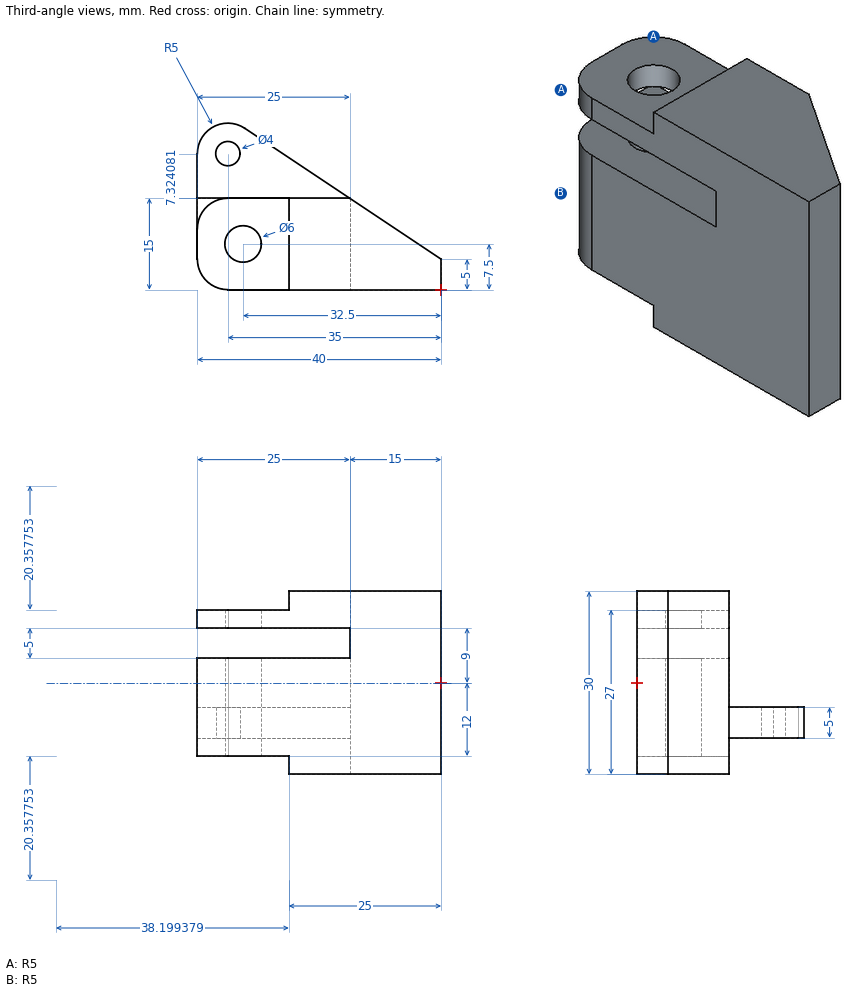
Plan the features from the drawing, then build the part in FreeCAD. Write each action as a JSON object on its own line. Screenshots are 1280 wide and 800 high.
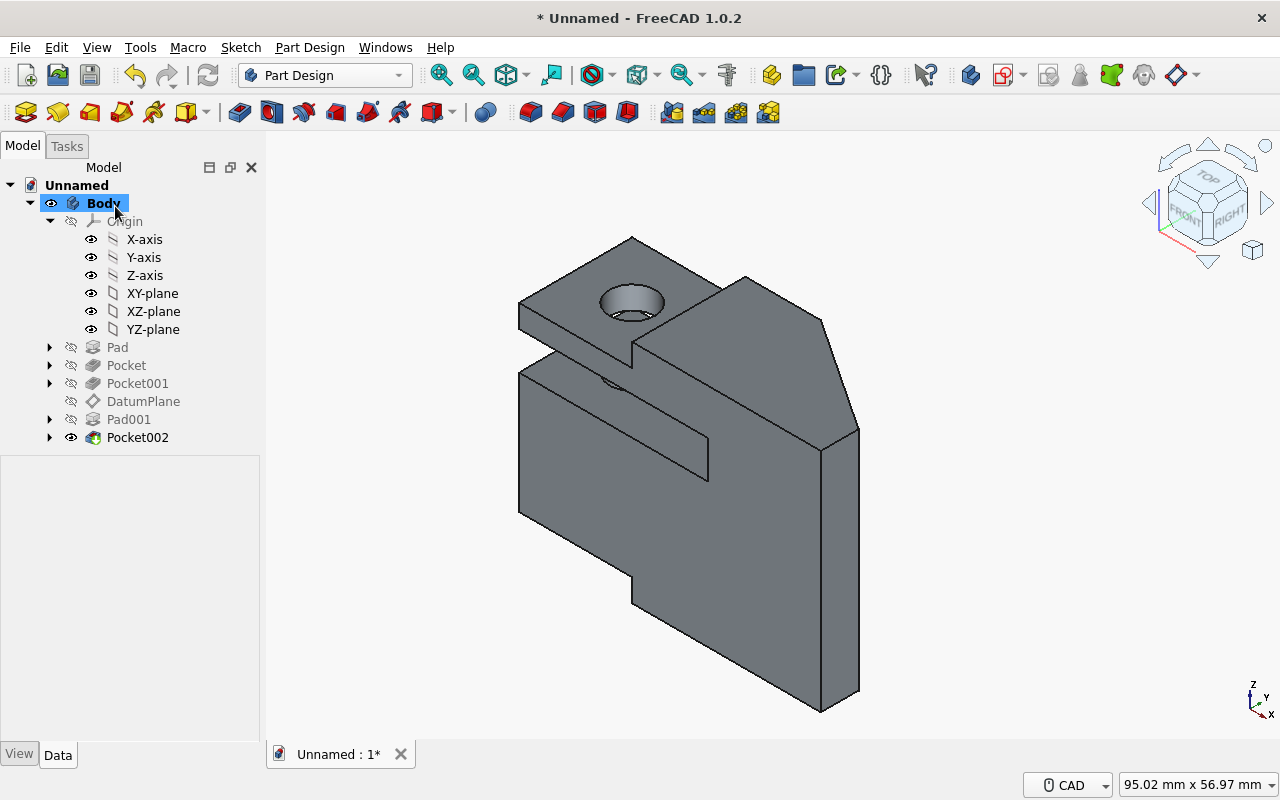
{"action": "key", "text": "2"}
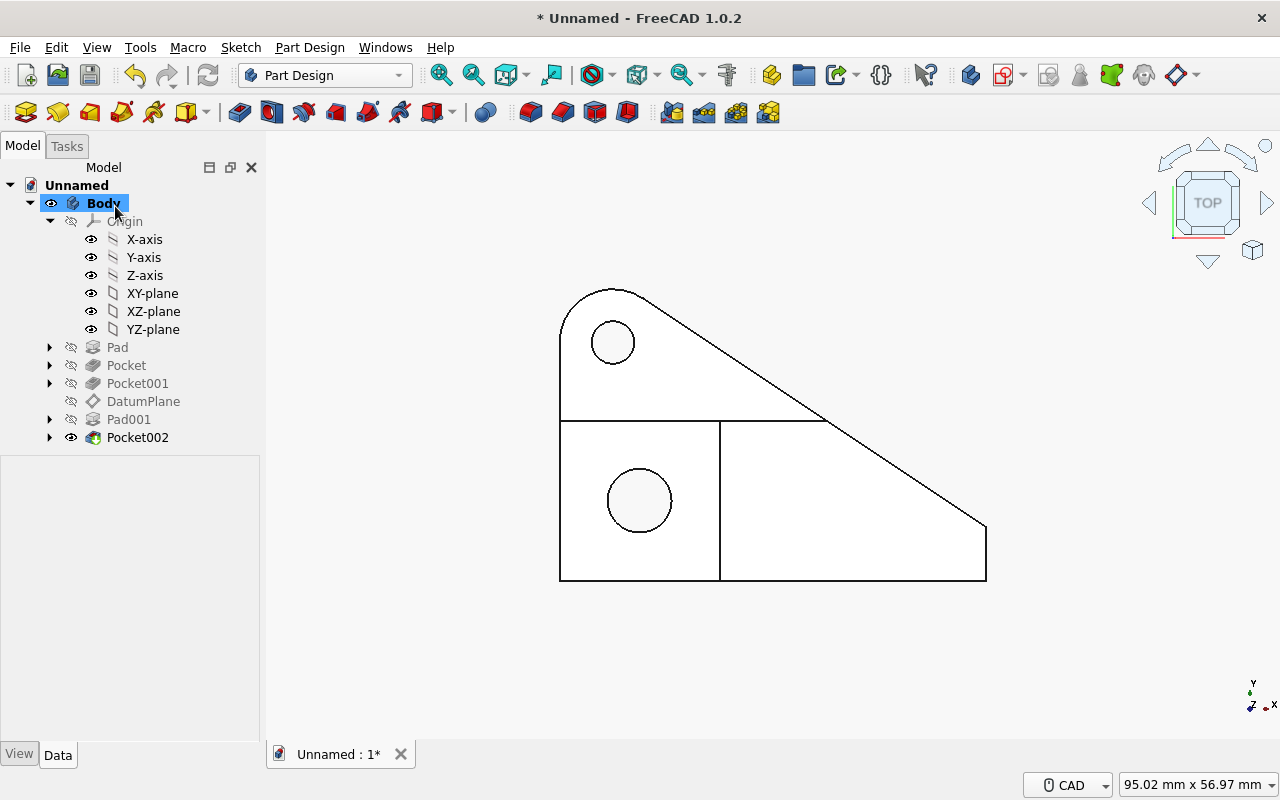
{"action": "key", "text": "0"}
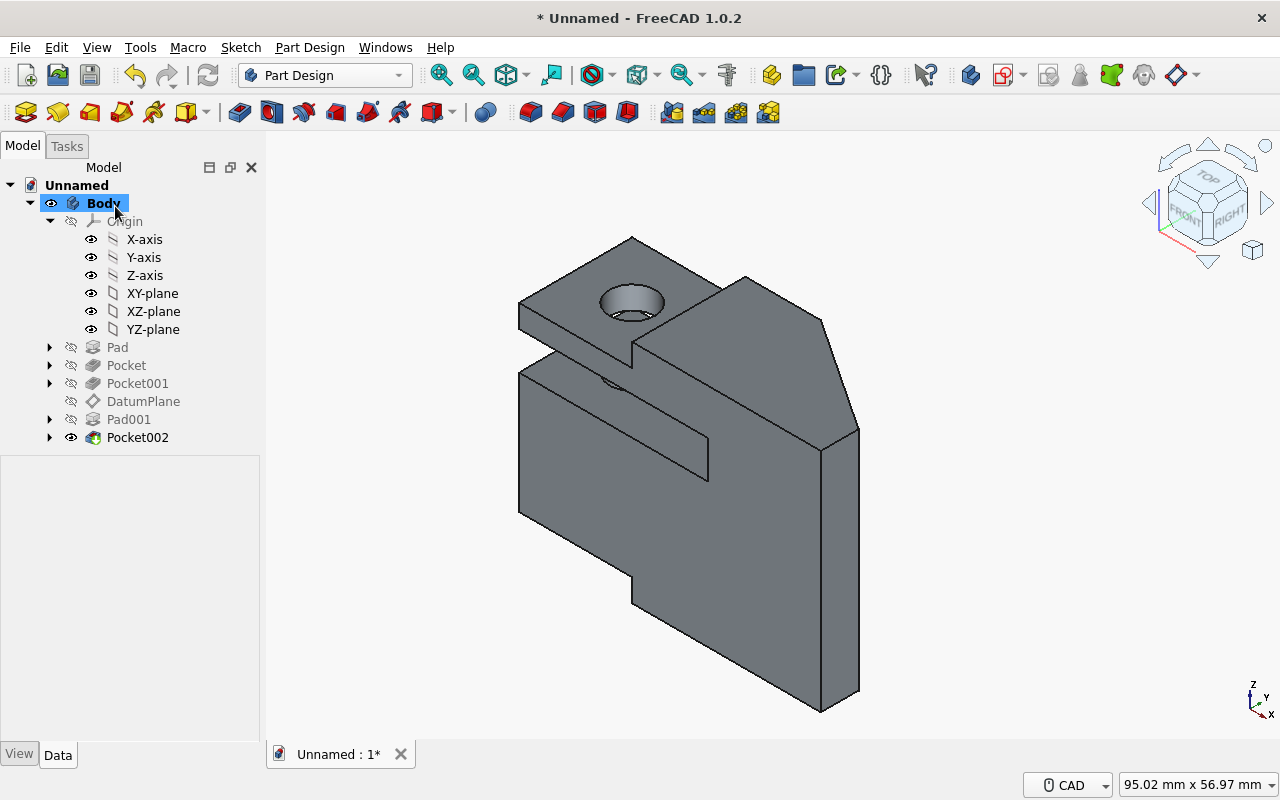
{"action": "key", "text": "1"}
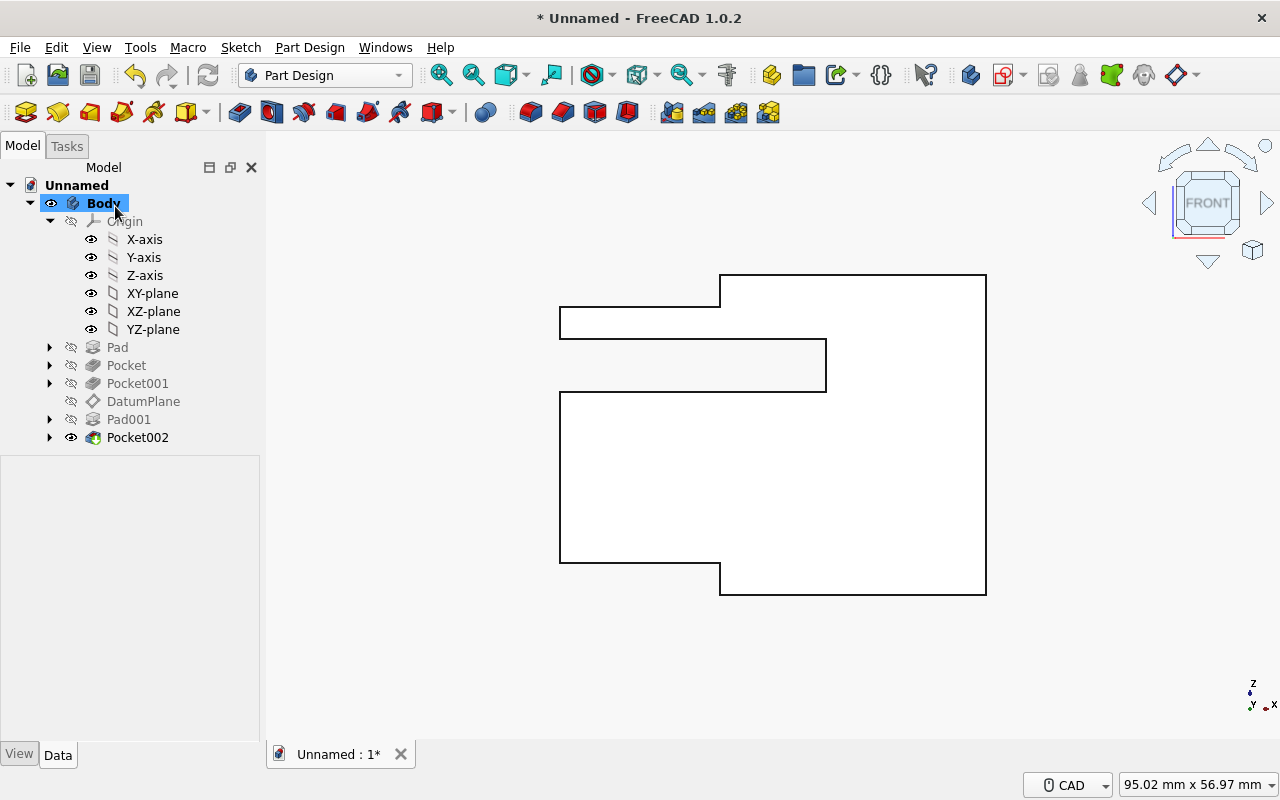
{"action": "left_click", "coordinate": [560, 322]}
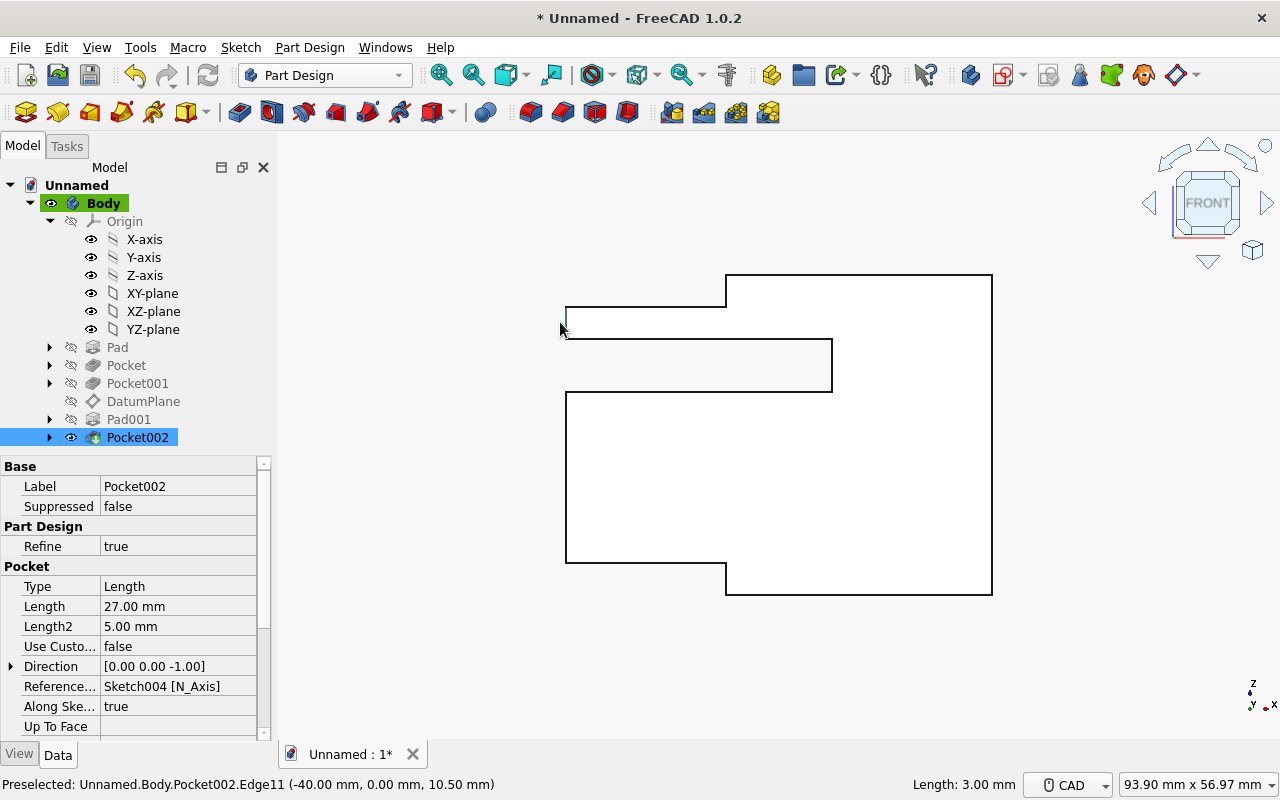
{"action": "key", "text": "3"}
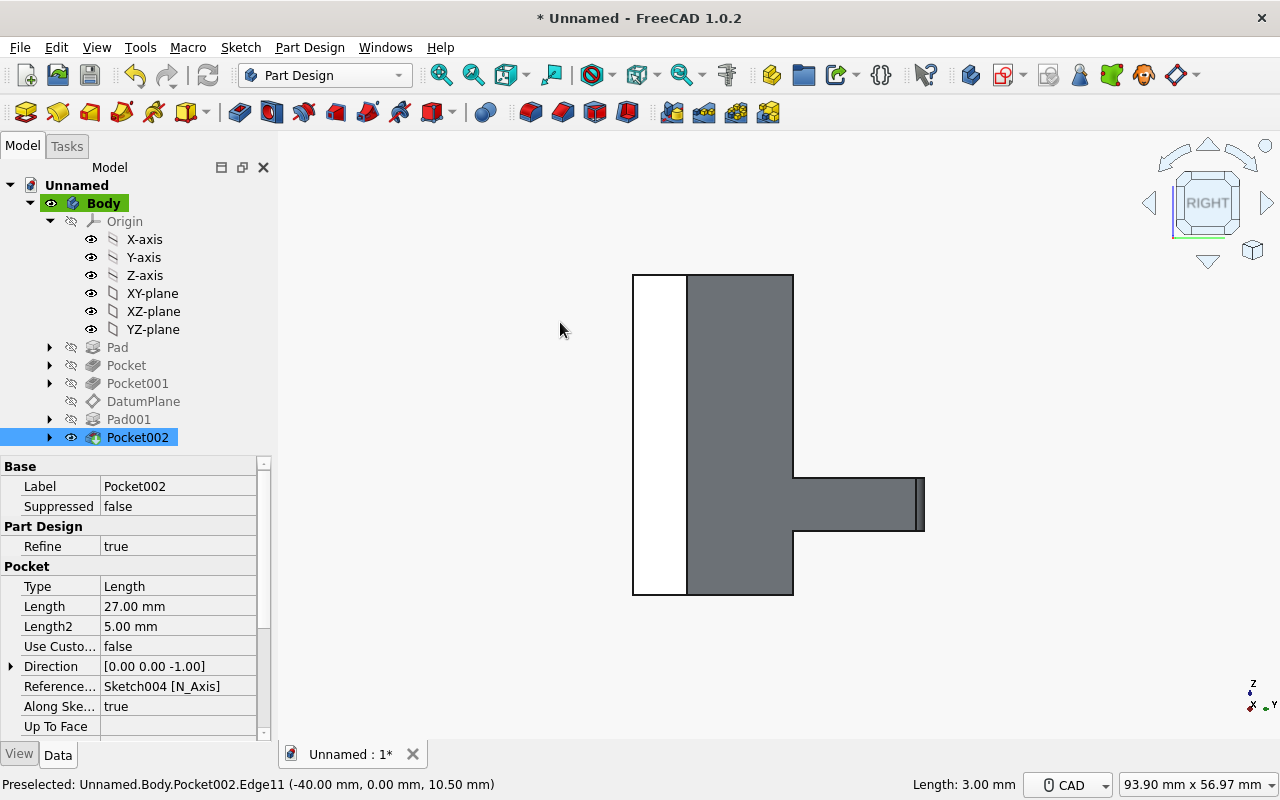
{"action": "key", "text": "5"}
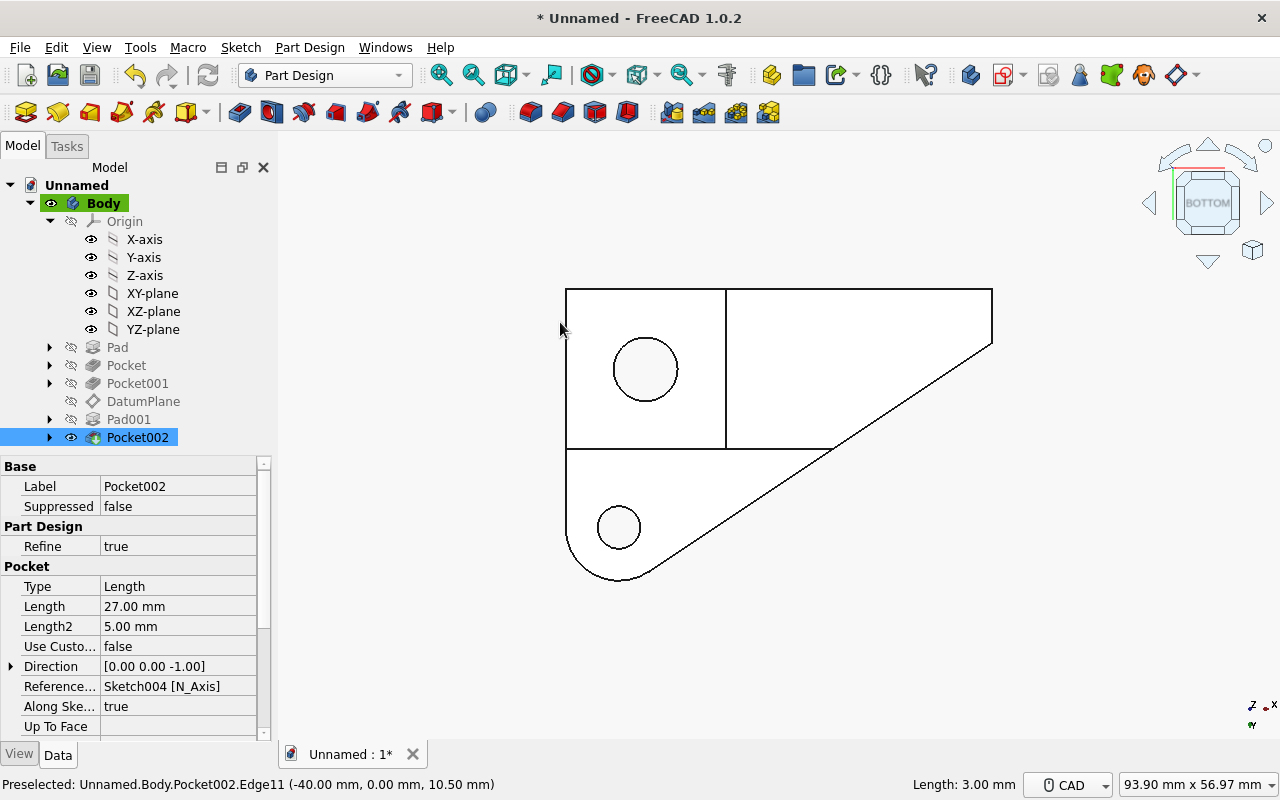
{"action": "key", "text": "4"}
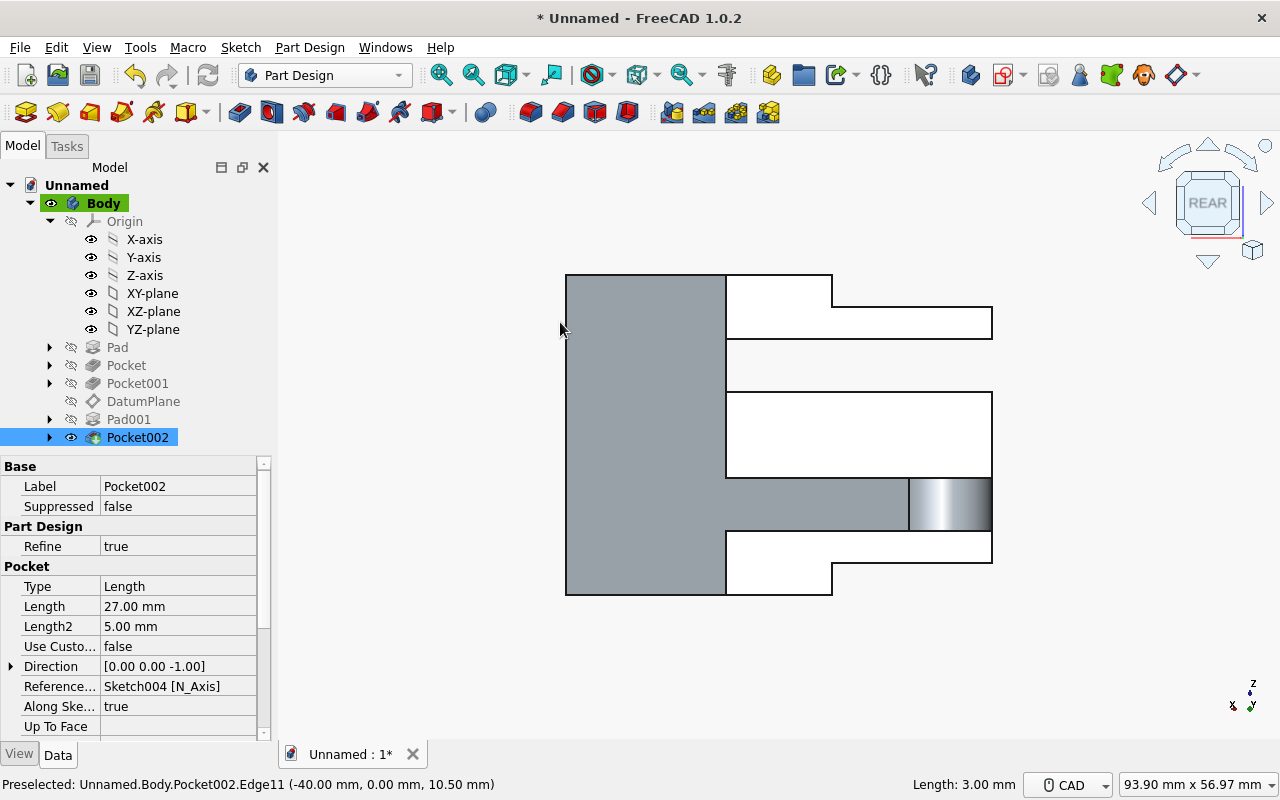
{"action": "left_click", "coordinate": [992, 322], "text": "ctrl"}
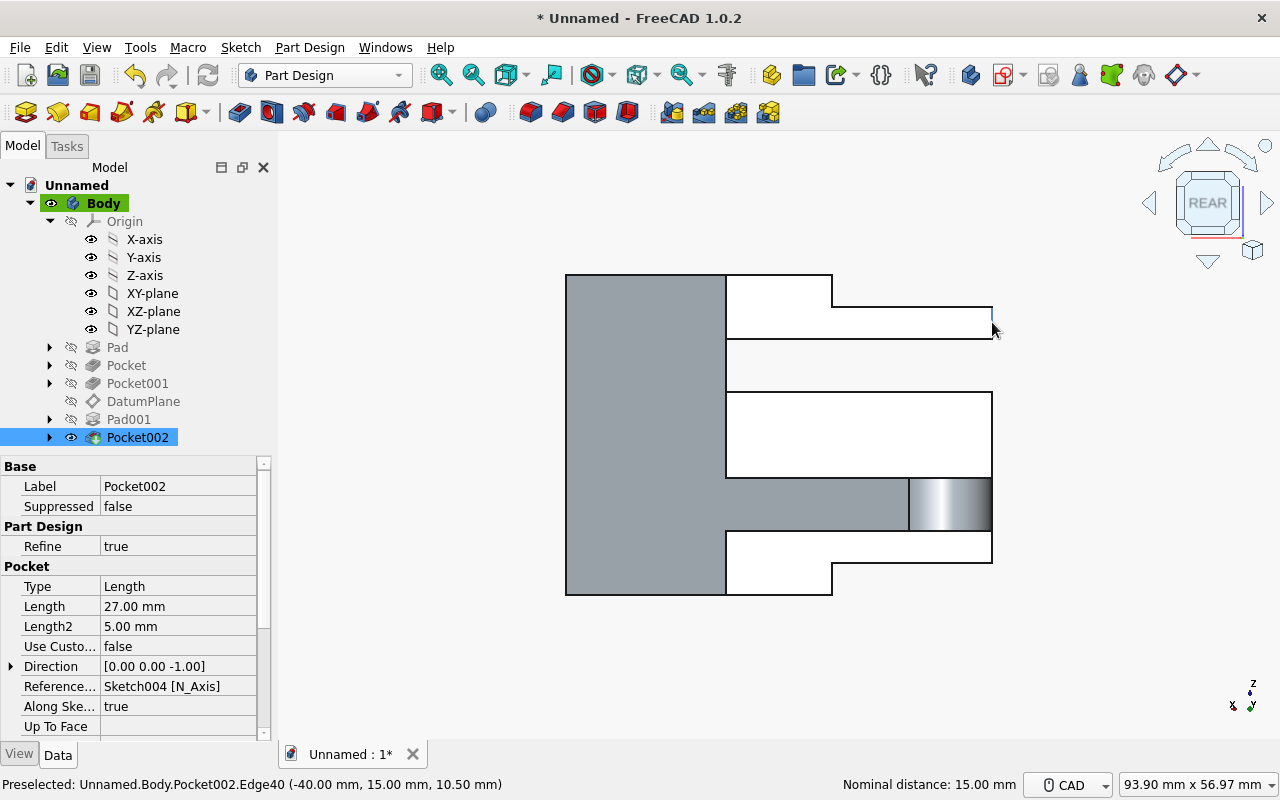
{"action": "left_click", "coordinate": [532, 112]}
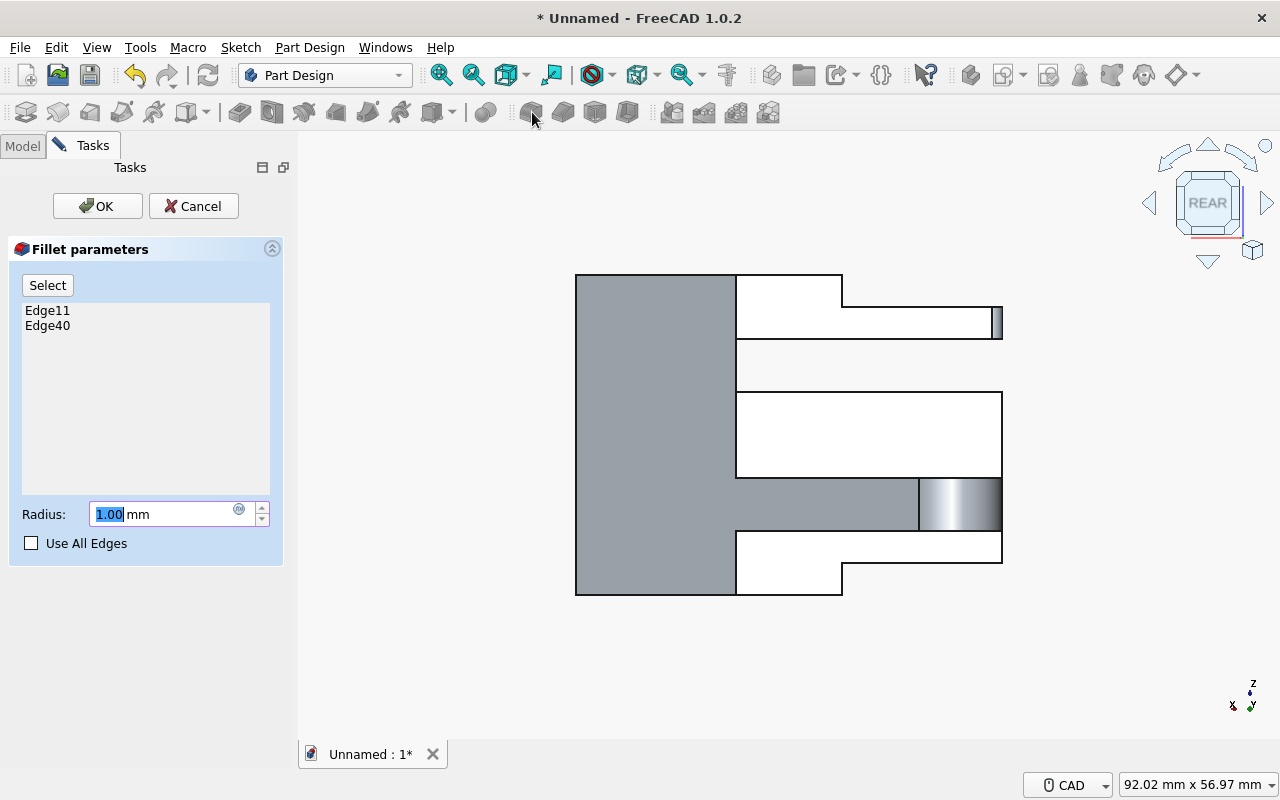
{"action": "type", "text": "5"}
{"action": "key", "text": "Tab"}